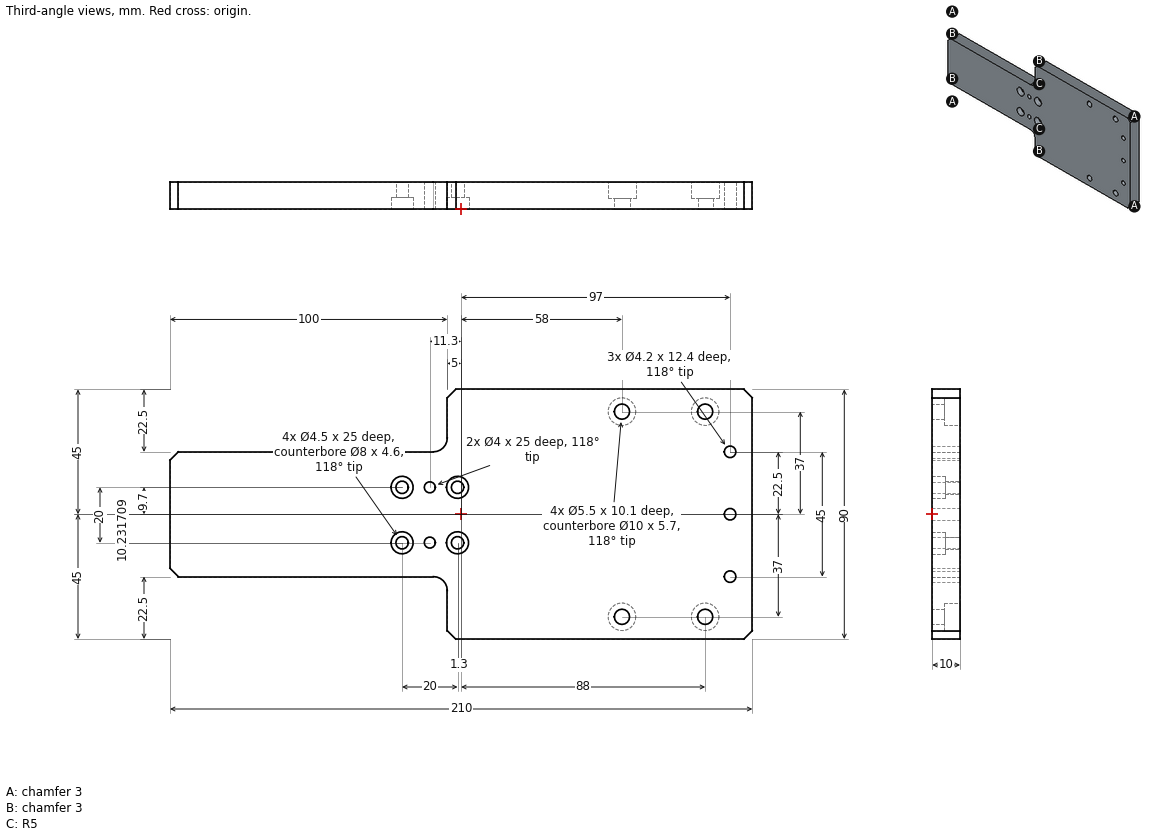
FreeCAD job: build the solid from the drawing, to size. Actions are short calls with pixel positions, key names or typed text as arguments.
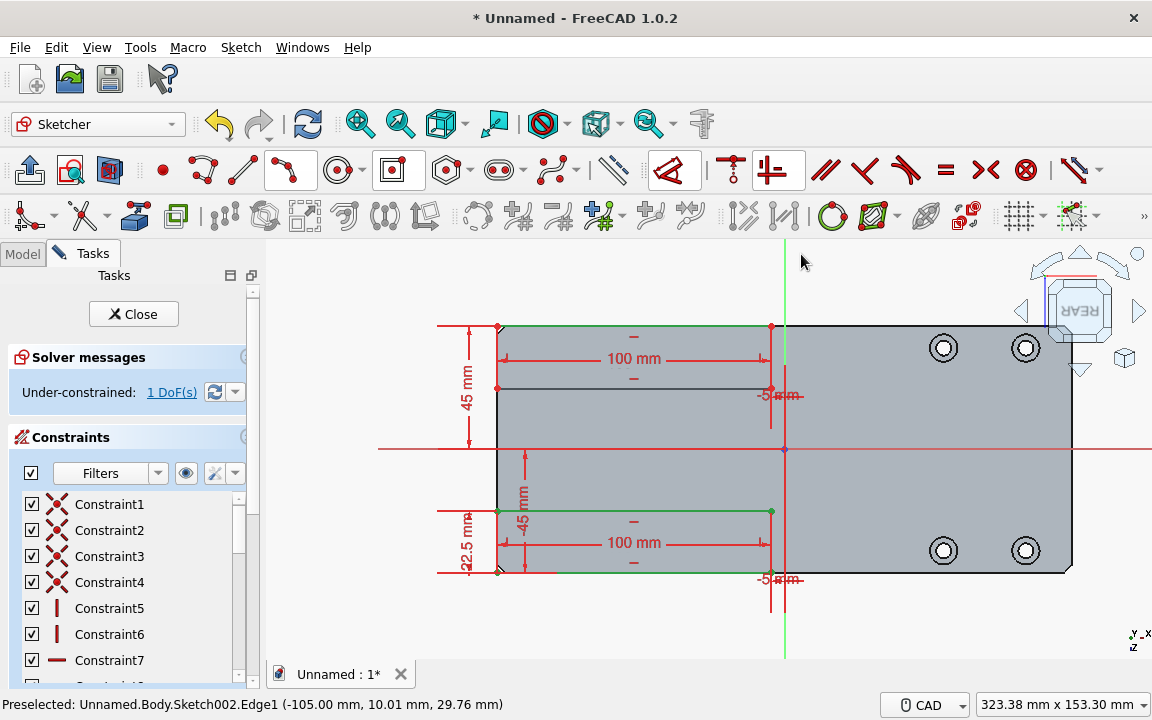
click(497, 345)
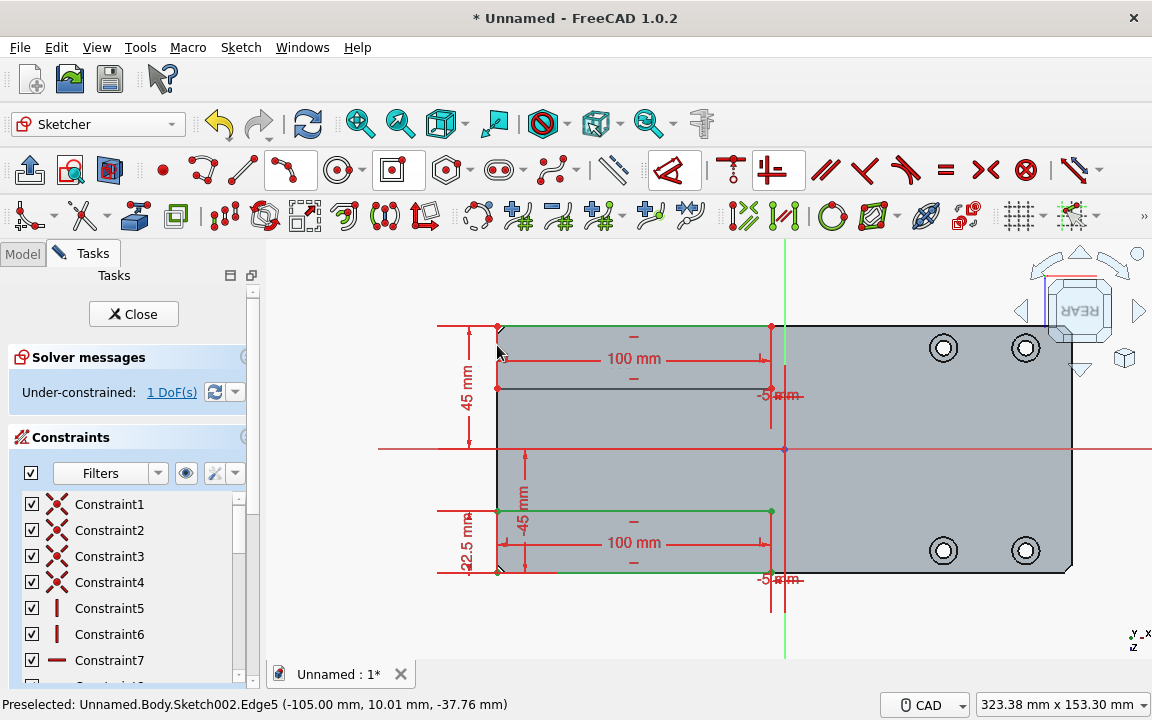
key(i)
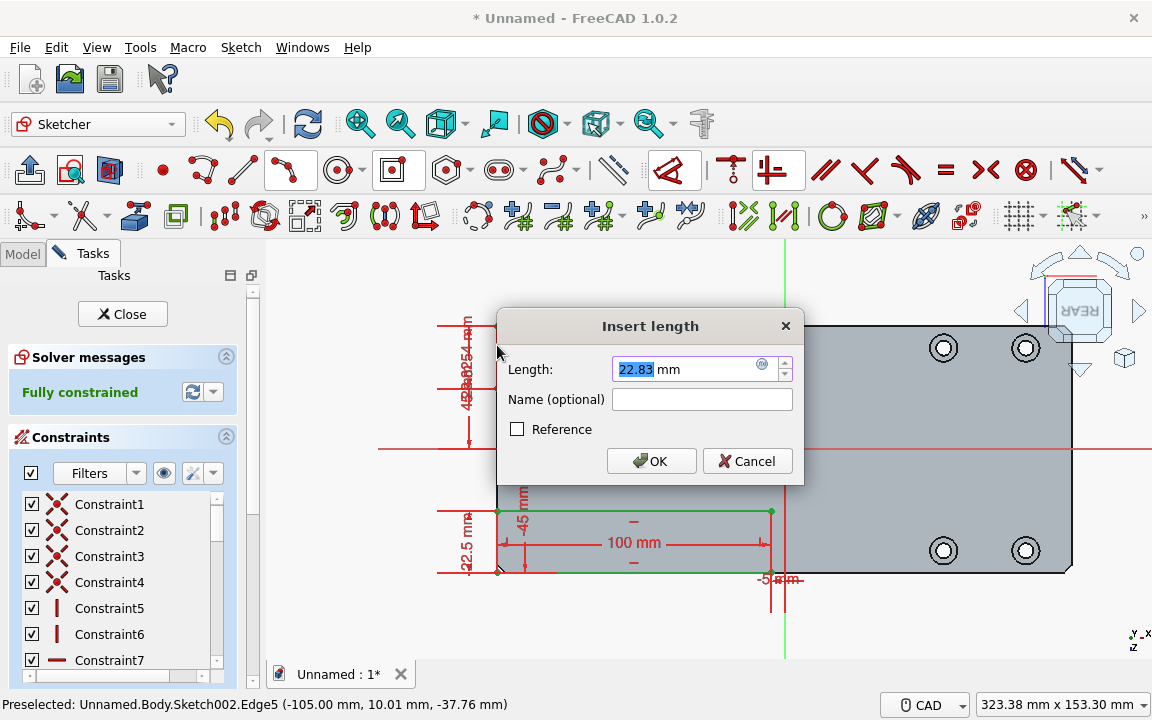
text(22.5)
key(Return)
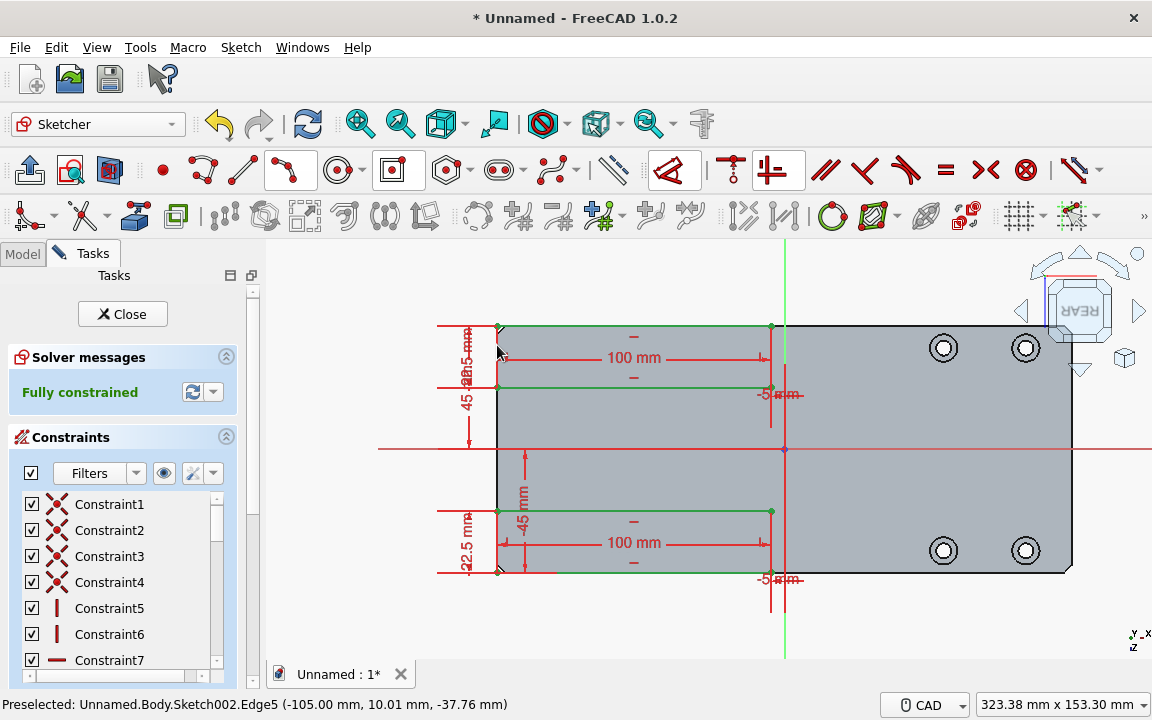
click(123, 314)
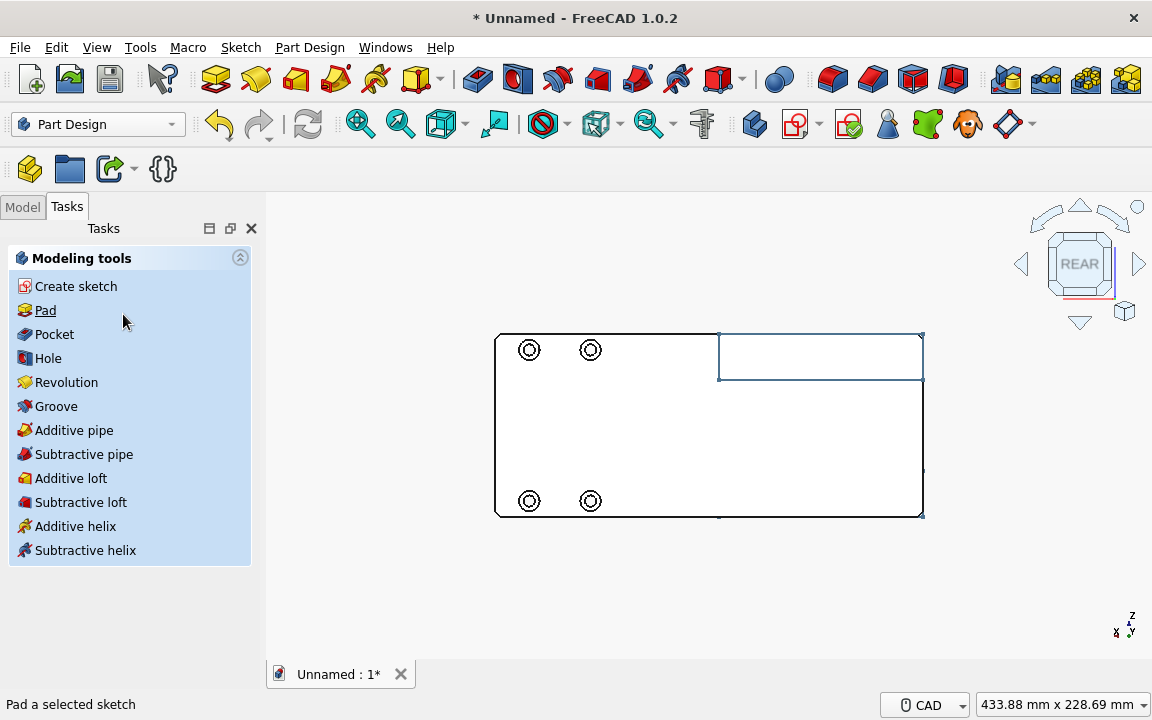
click(478, 80)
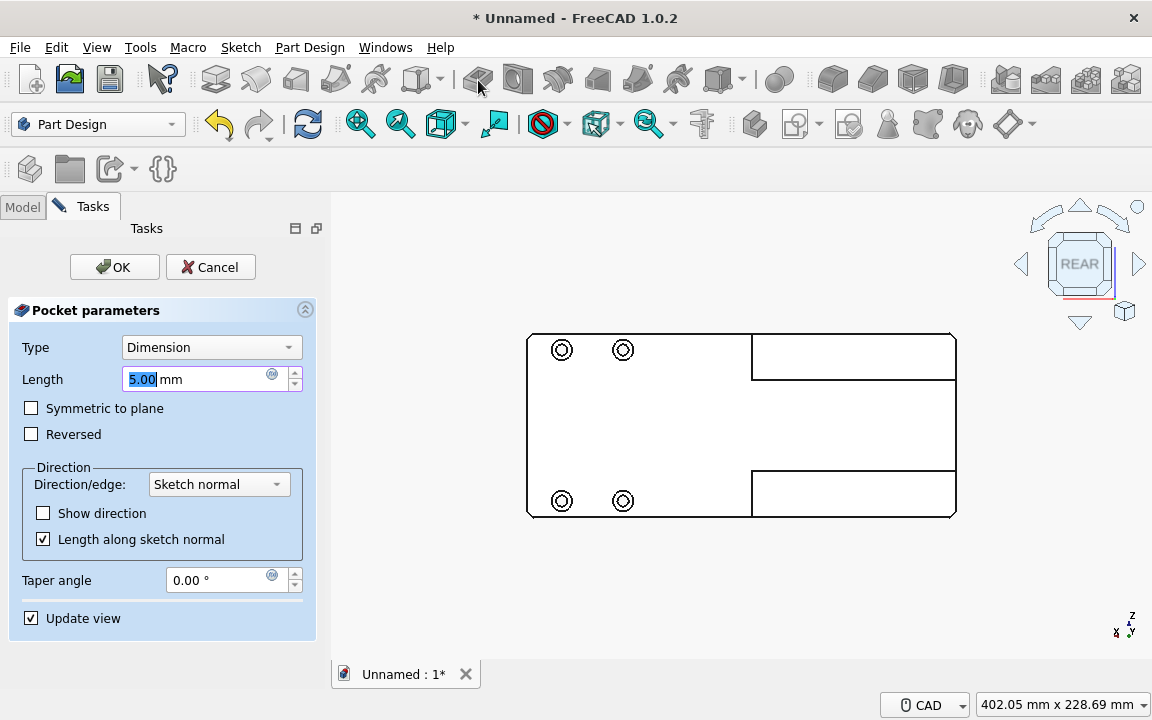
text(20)
key(Tab)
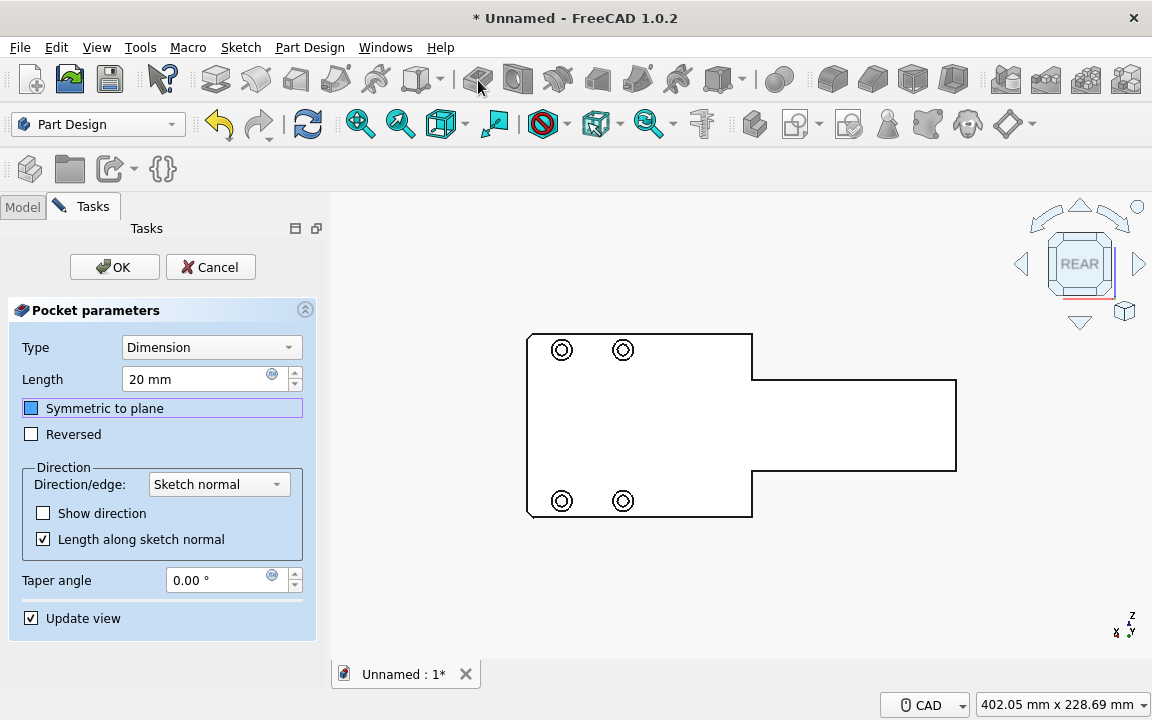
click(115, 267)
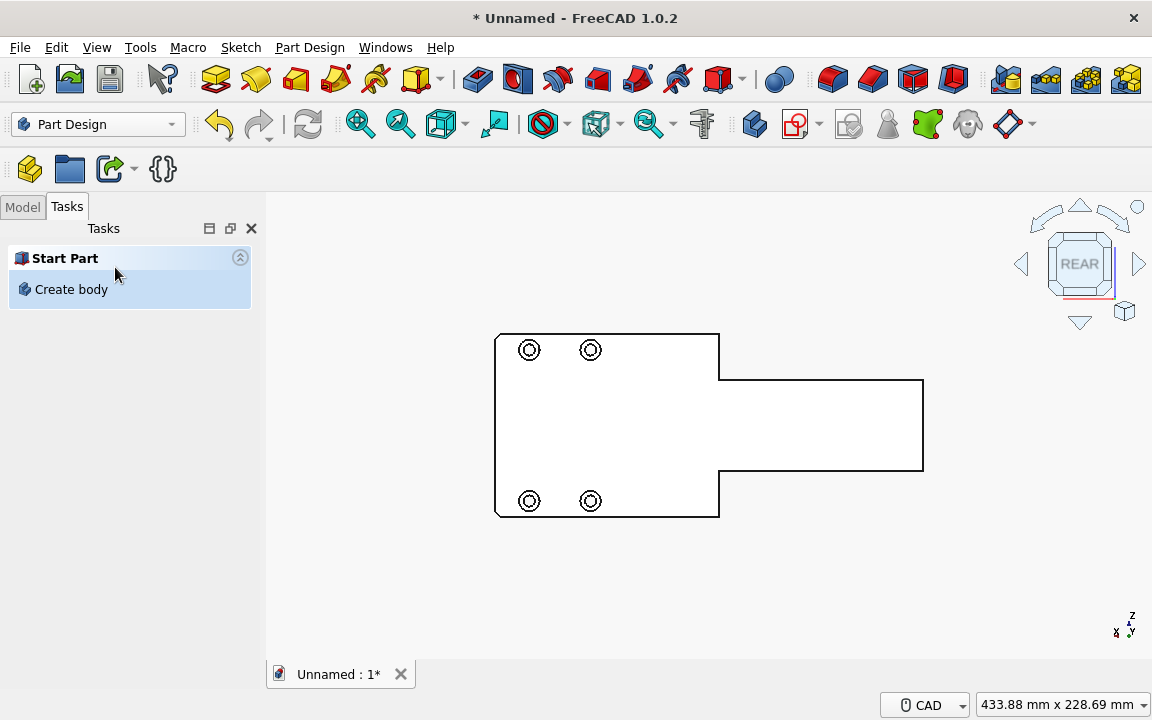
scroll(923, 379, up, 4)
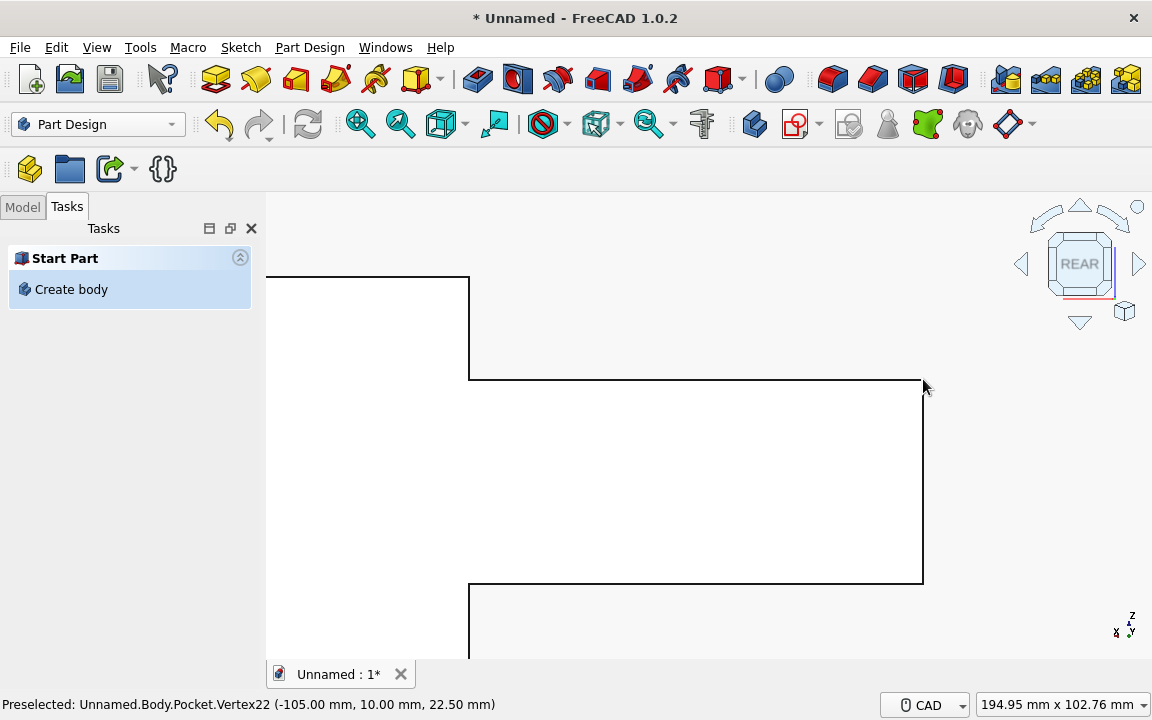
click(362, 124)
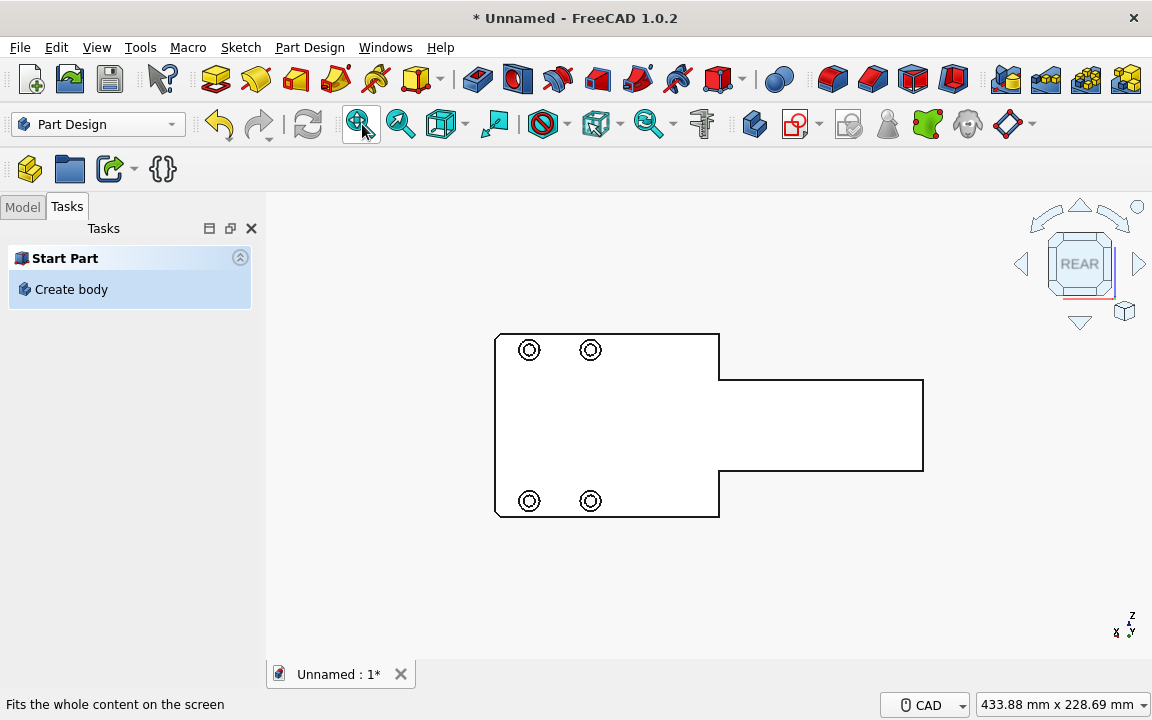
key(0)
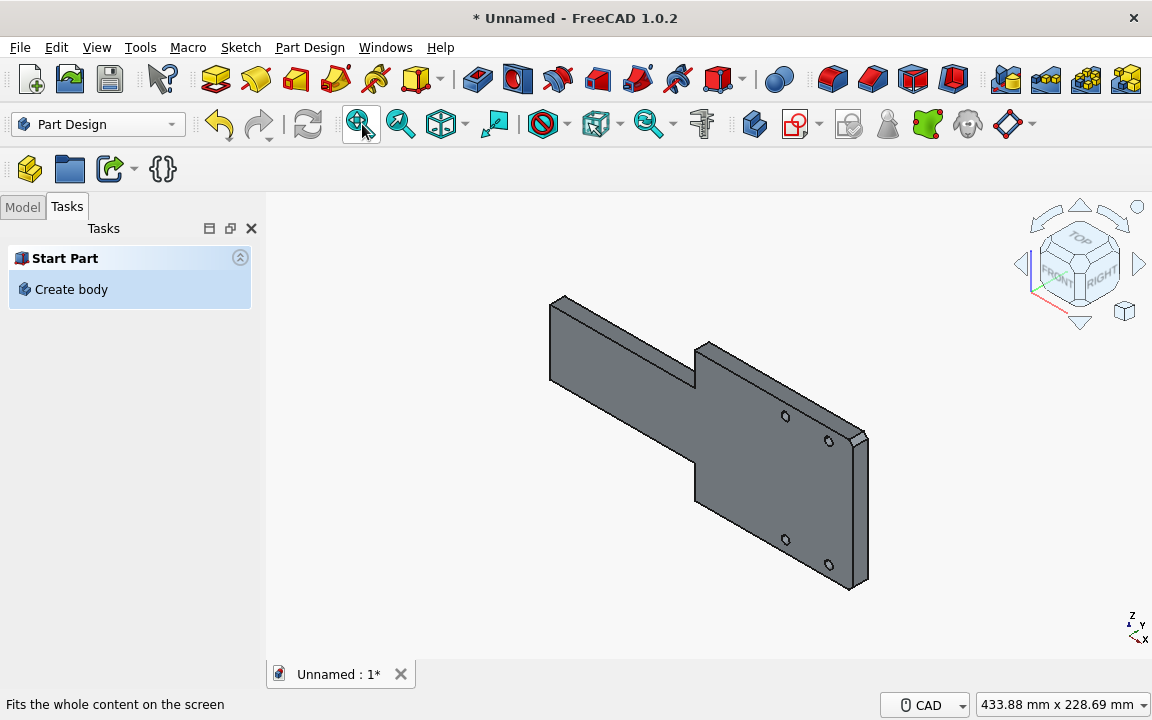
scroll(557, 299, up, 4)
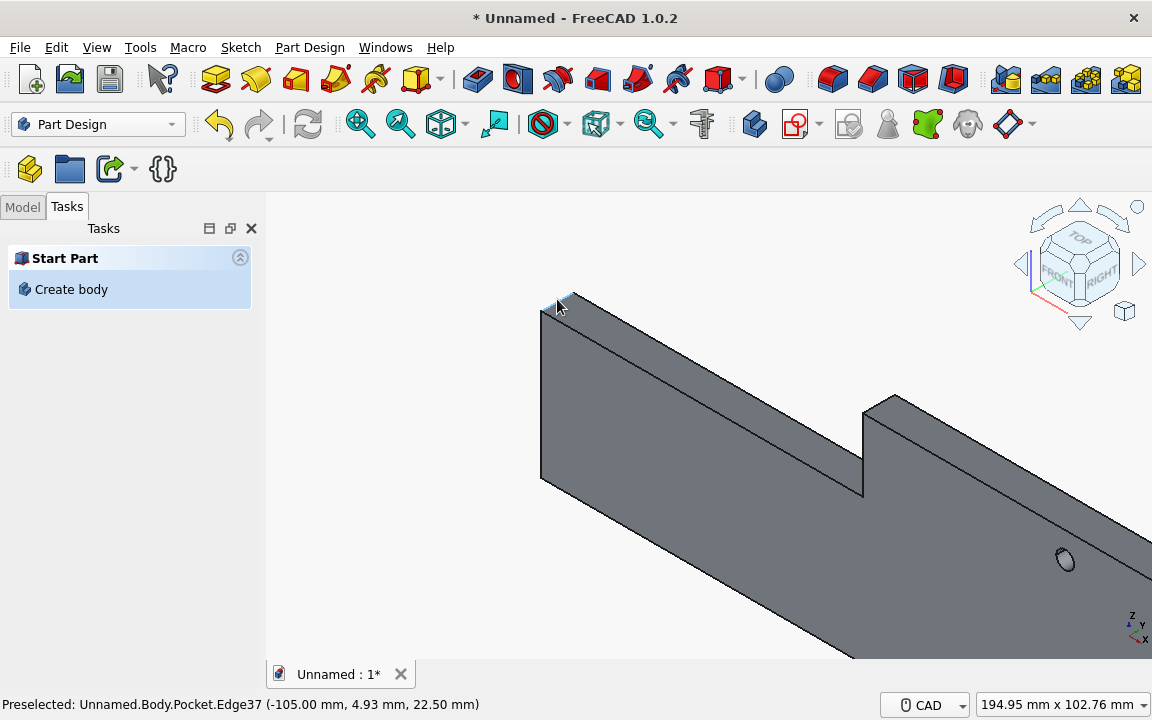
click(362, 124)